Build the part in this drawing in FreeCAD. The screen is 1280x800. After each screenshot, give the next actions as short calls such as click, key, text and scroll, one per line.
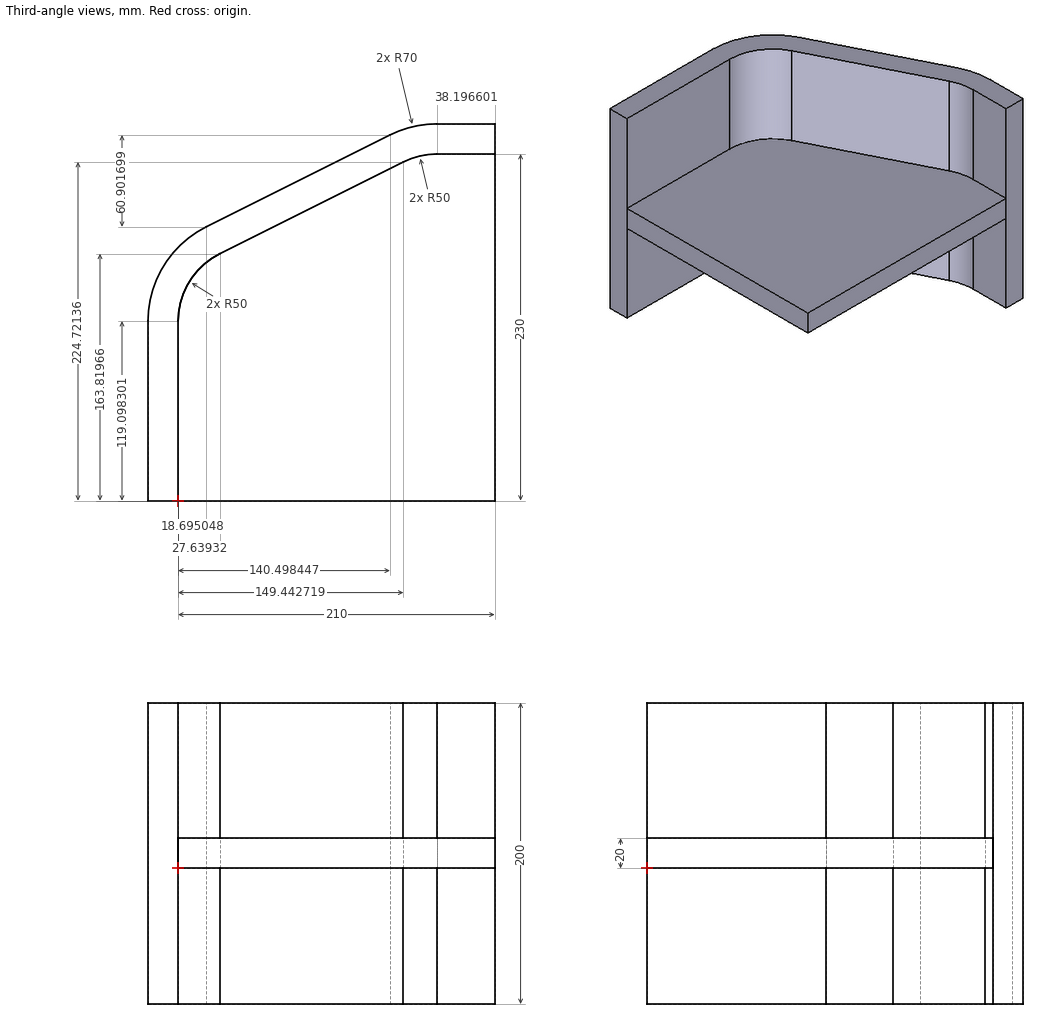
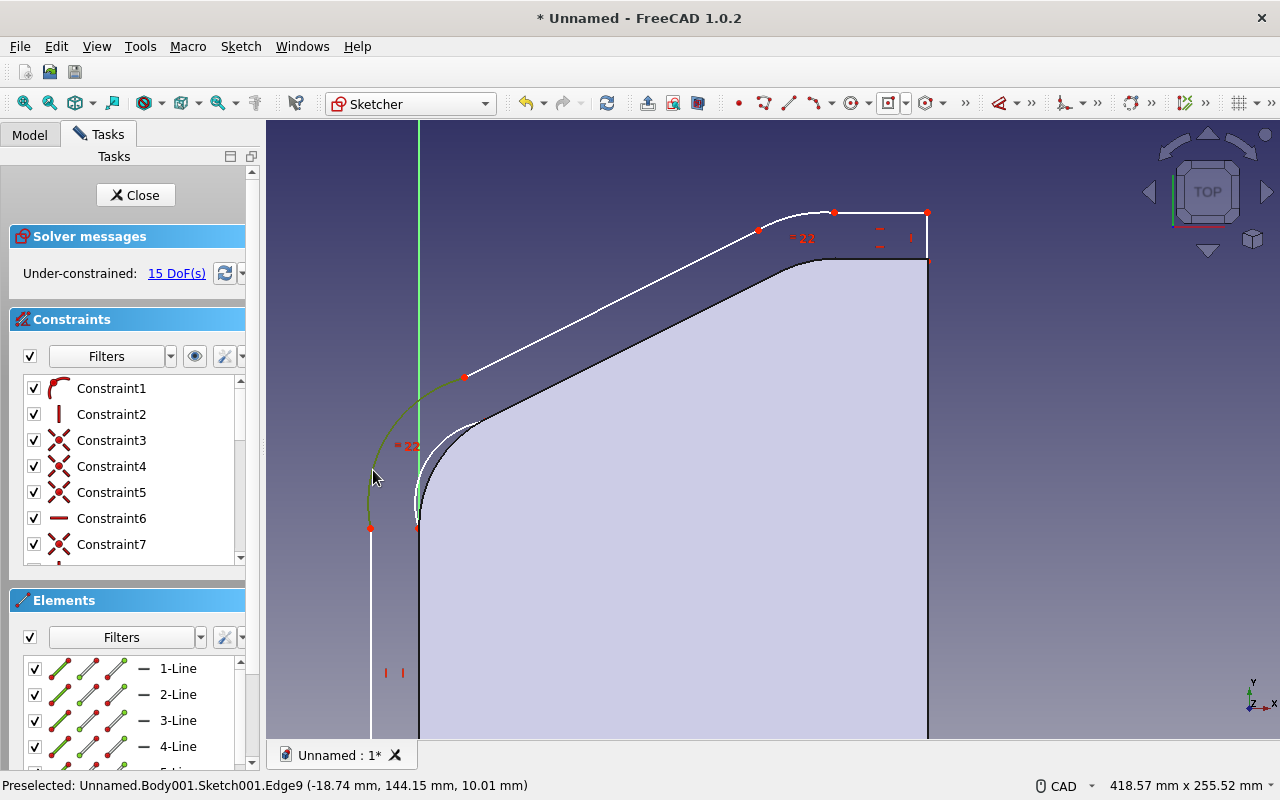
click(811, 213)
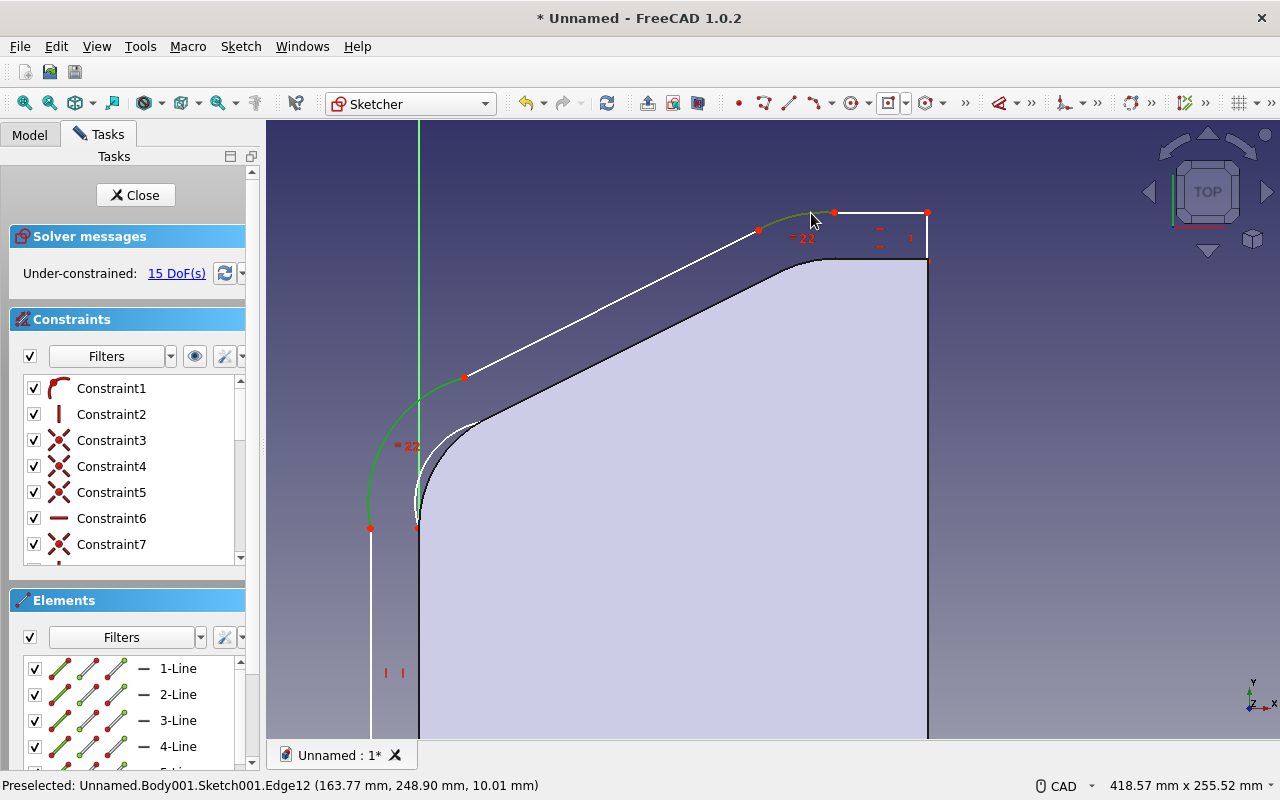
key(e)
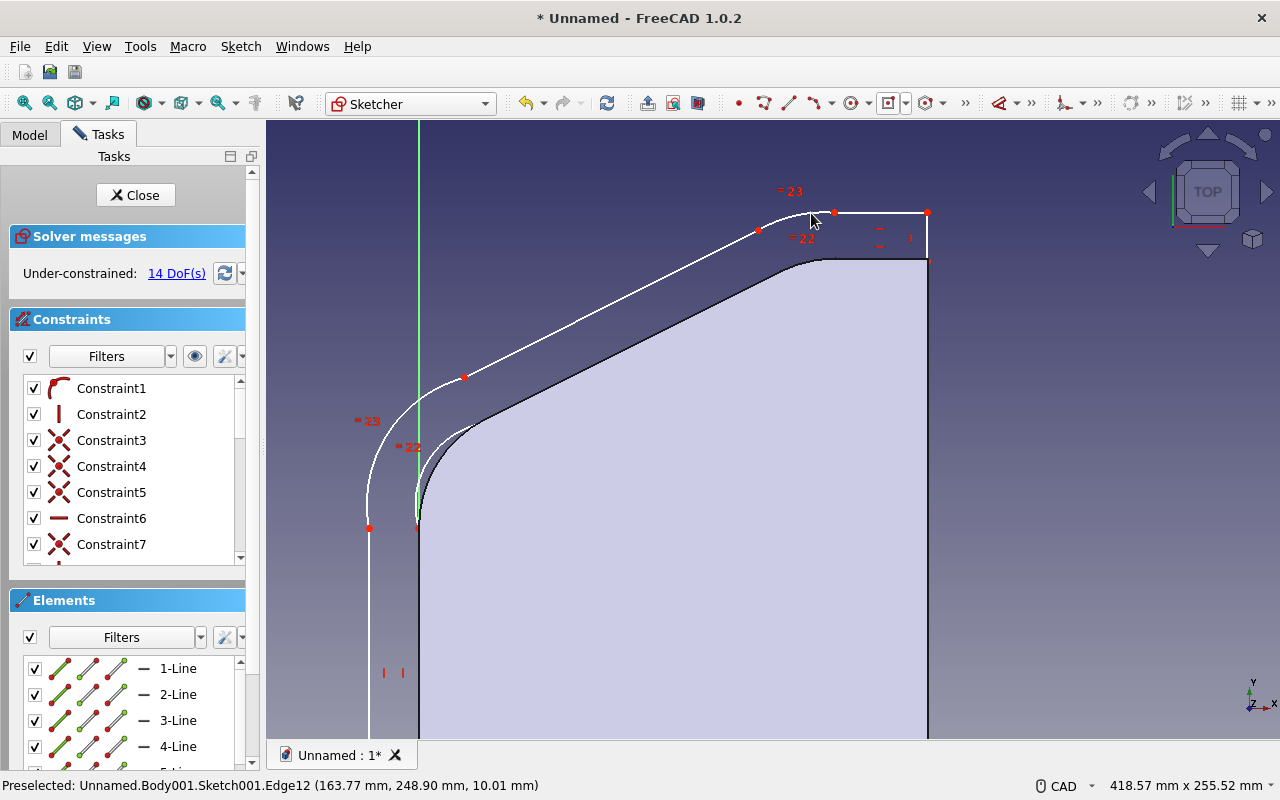
click(998, 104)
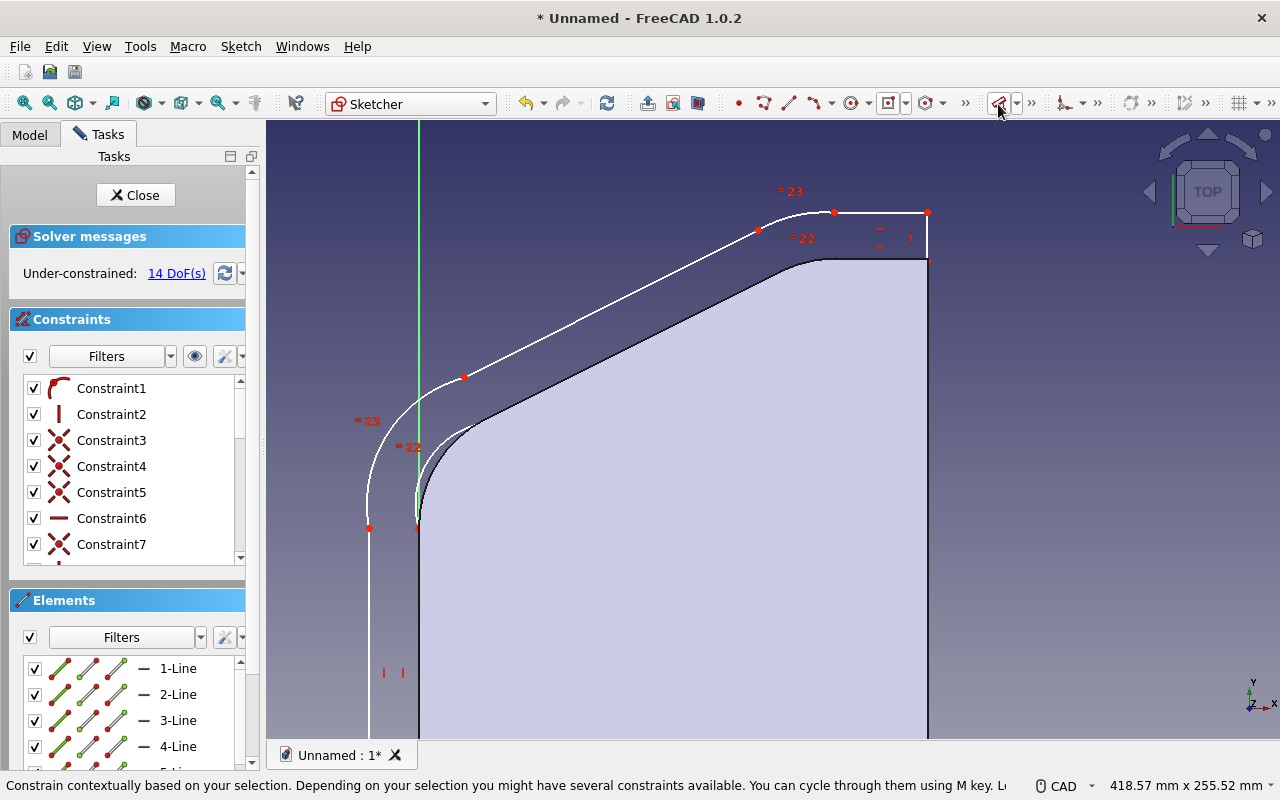
click(372, 470)
click(341, 462)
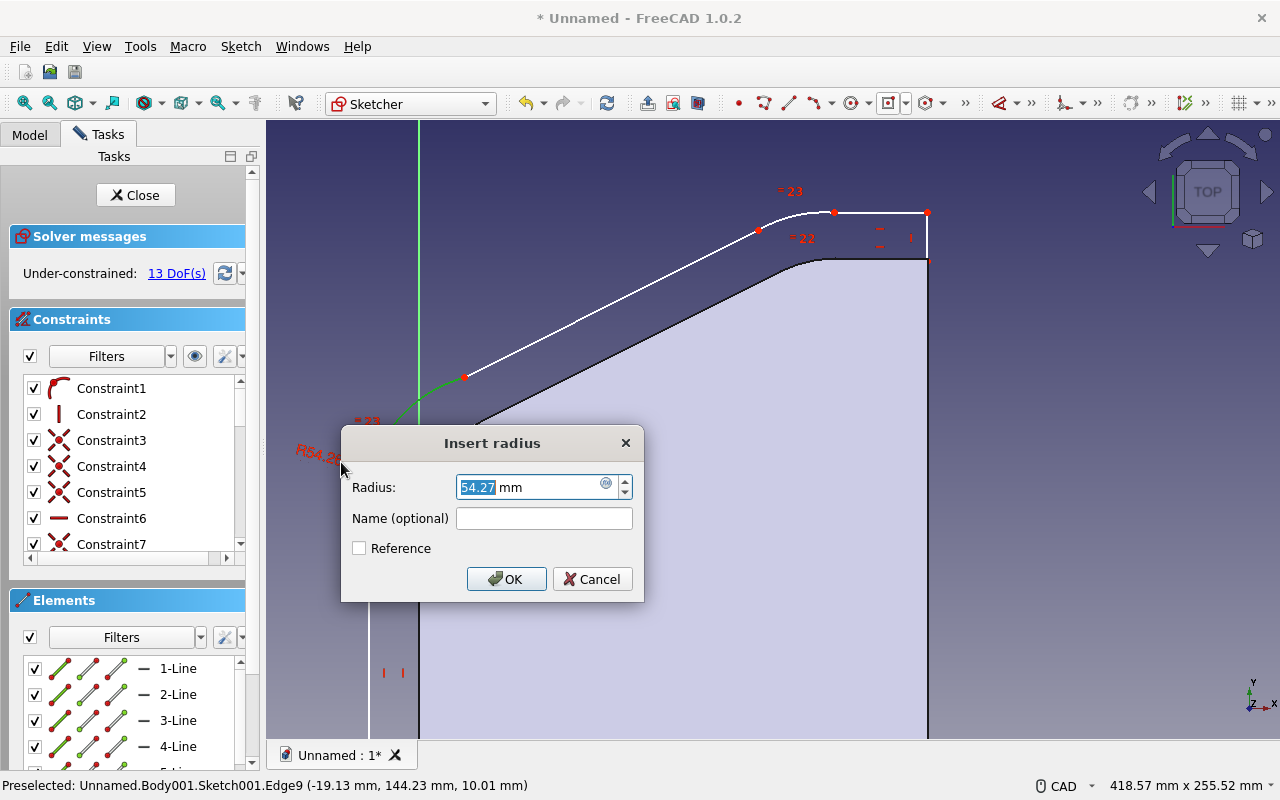
text(70)
key(Return)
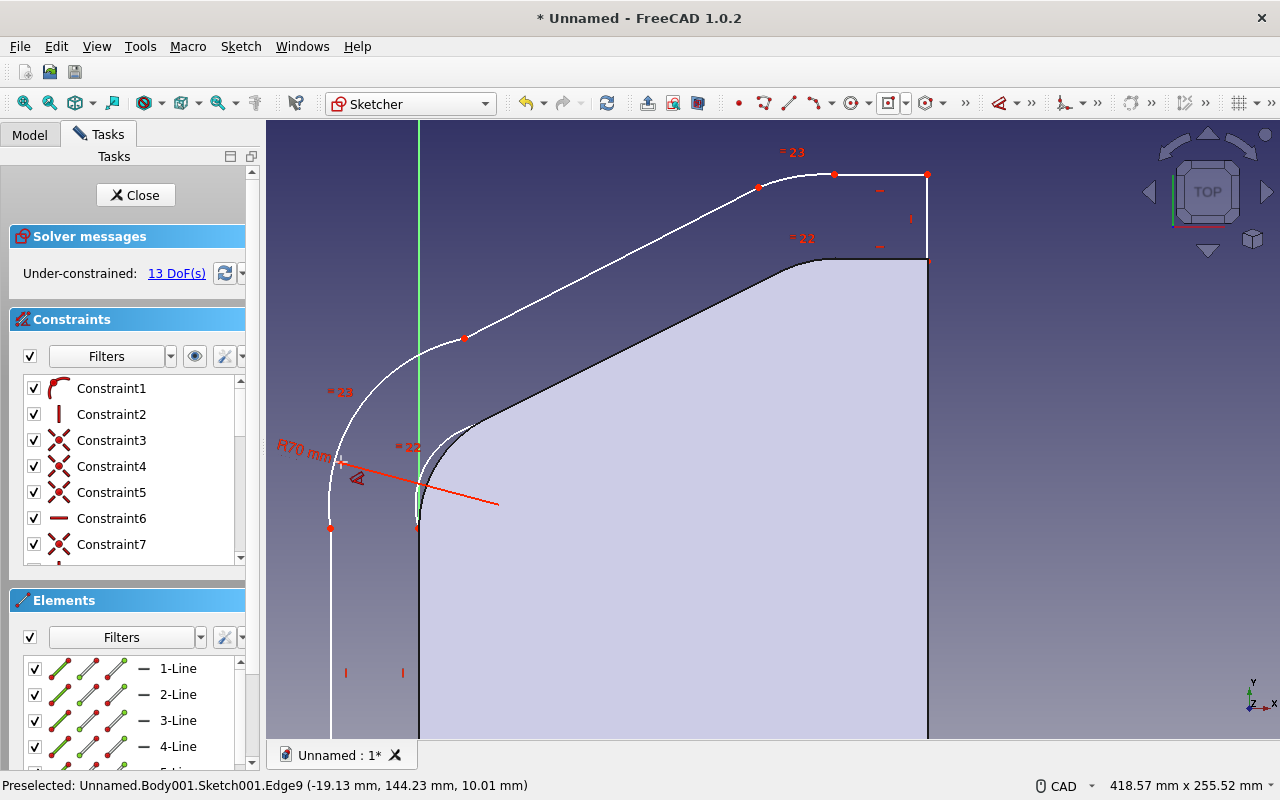
click(447, 440)
click(479, 392)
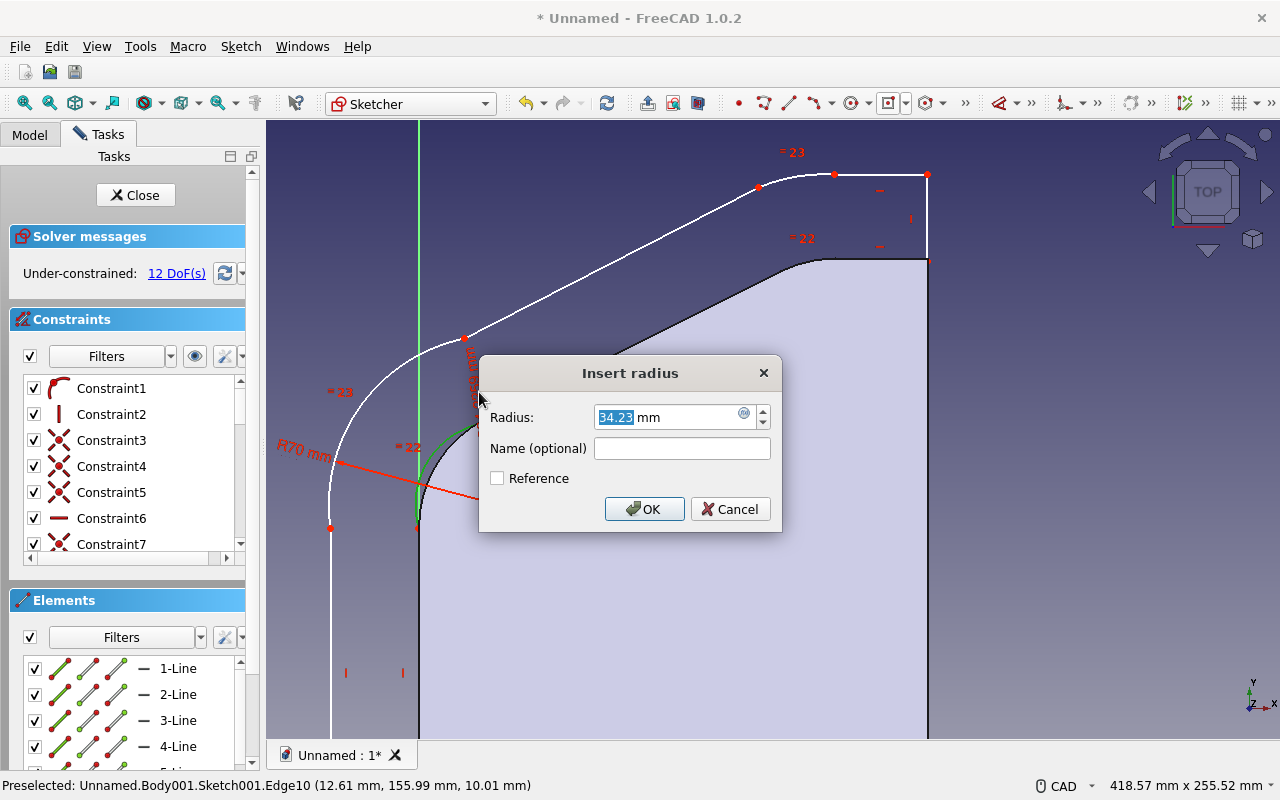
text(50)
key(Return)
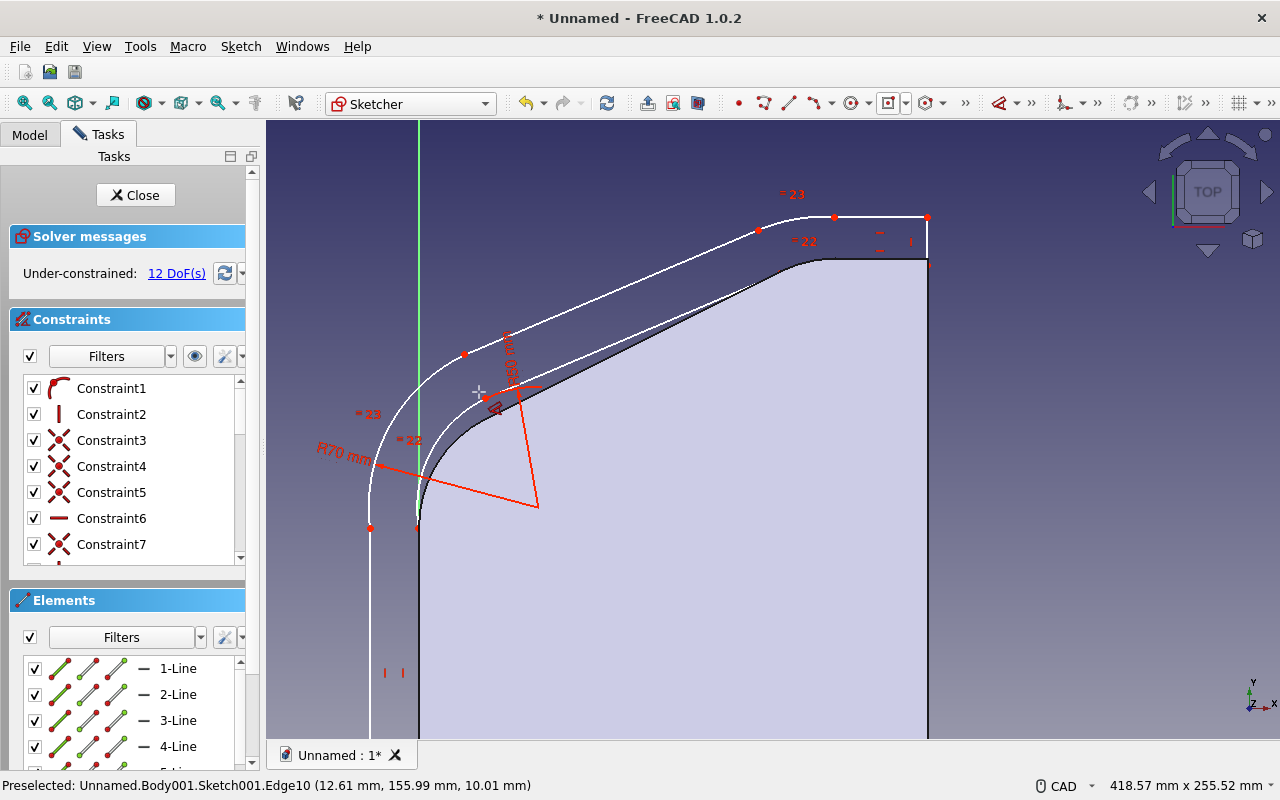
click(835, 266)
click(385, 488)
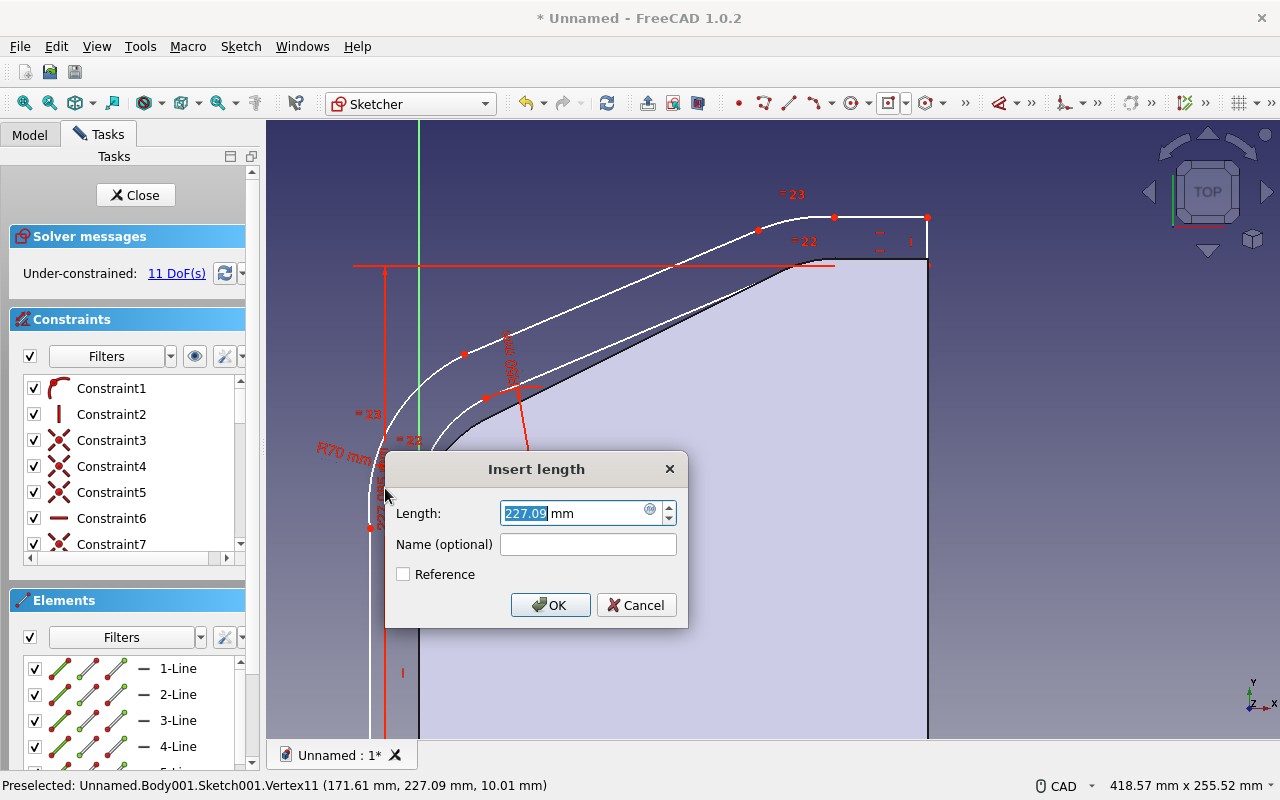
text(230)
key(Return)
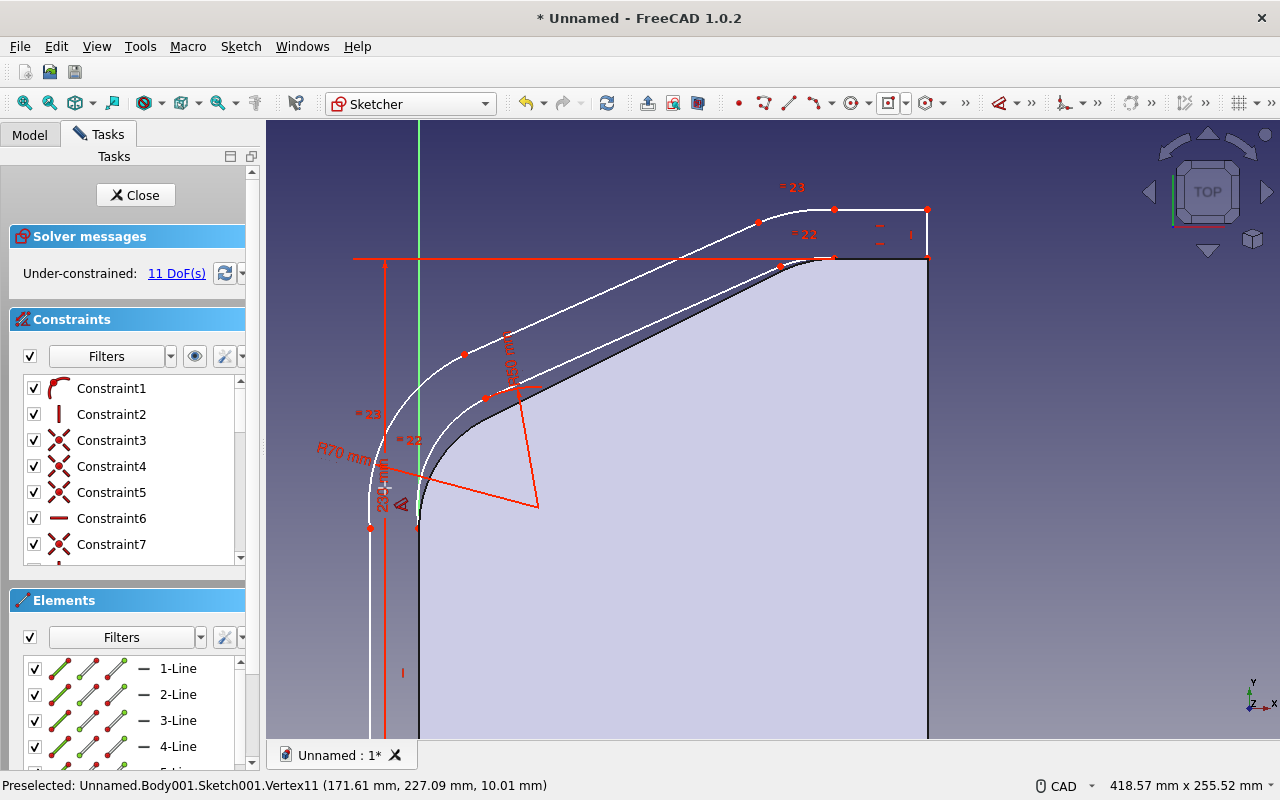
click(927, 259)
click(673, 225)